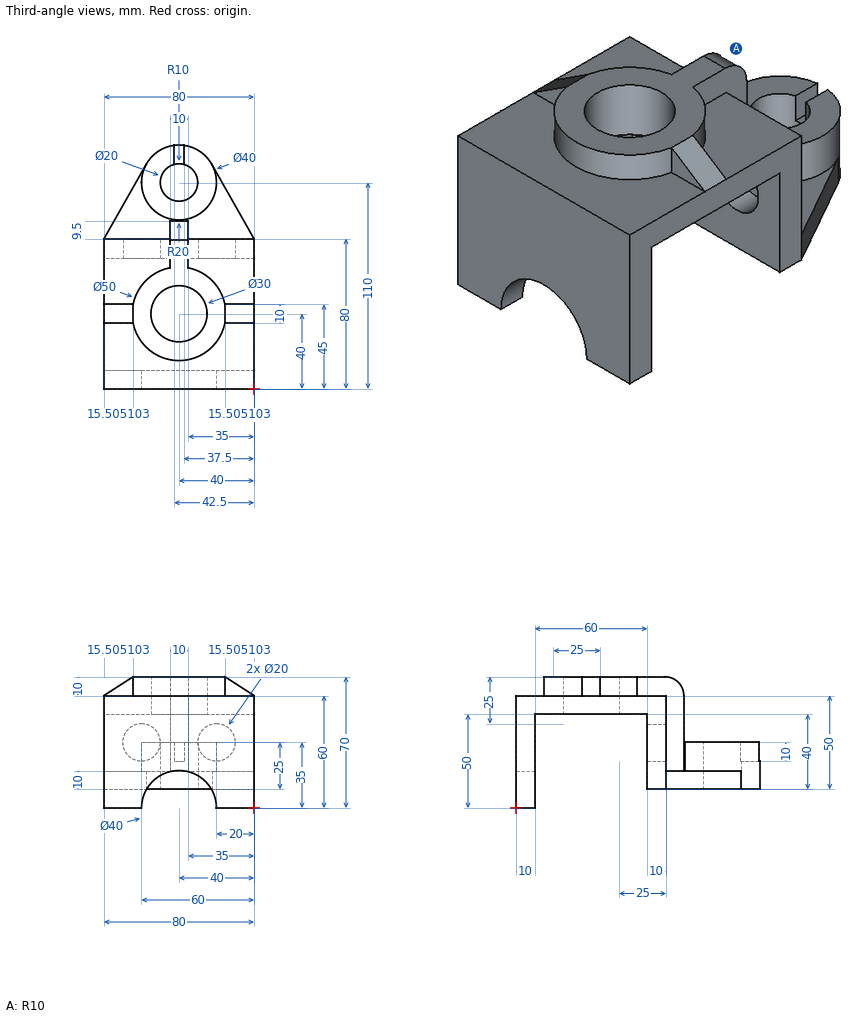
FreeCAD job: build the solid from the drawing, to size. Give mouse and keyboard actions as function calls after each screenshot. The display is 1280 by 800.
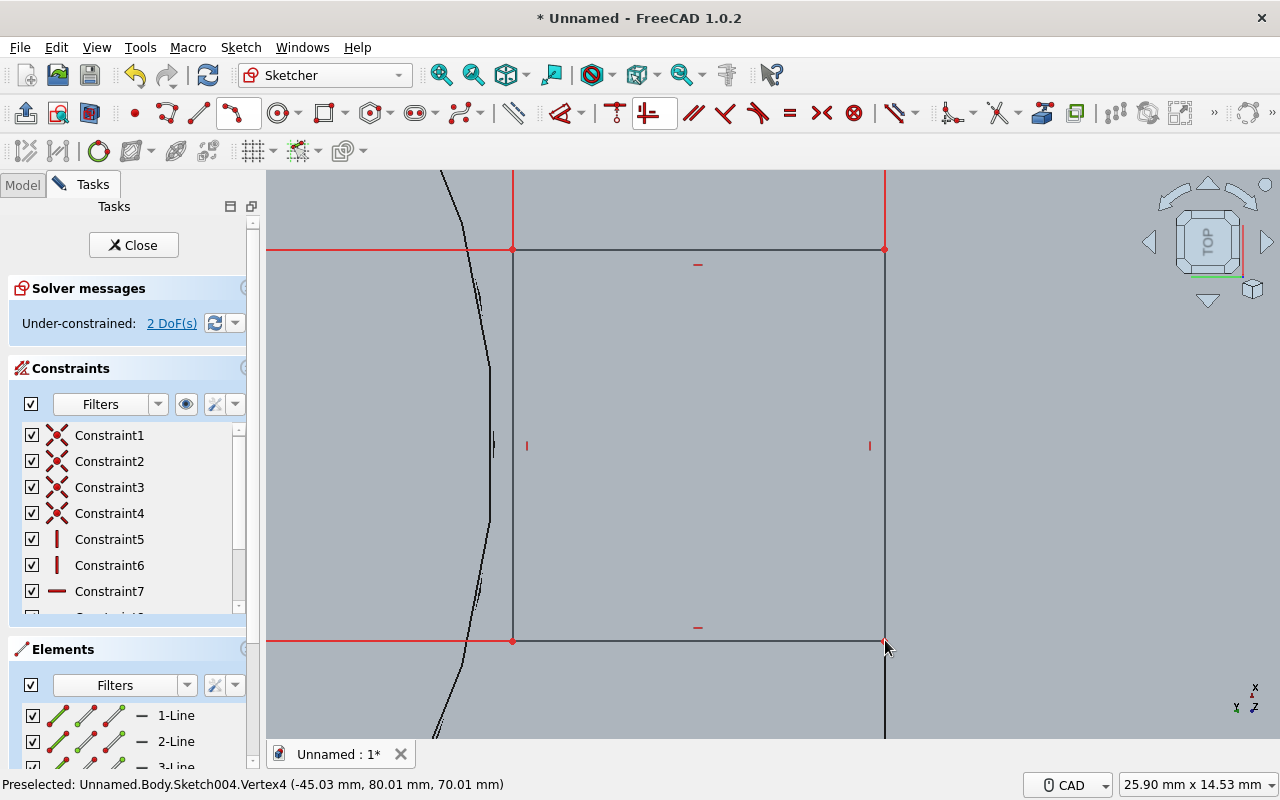
click(560, 114)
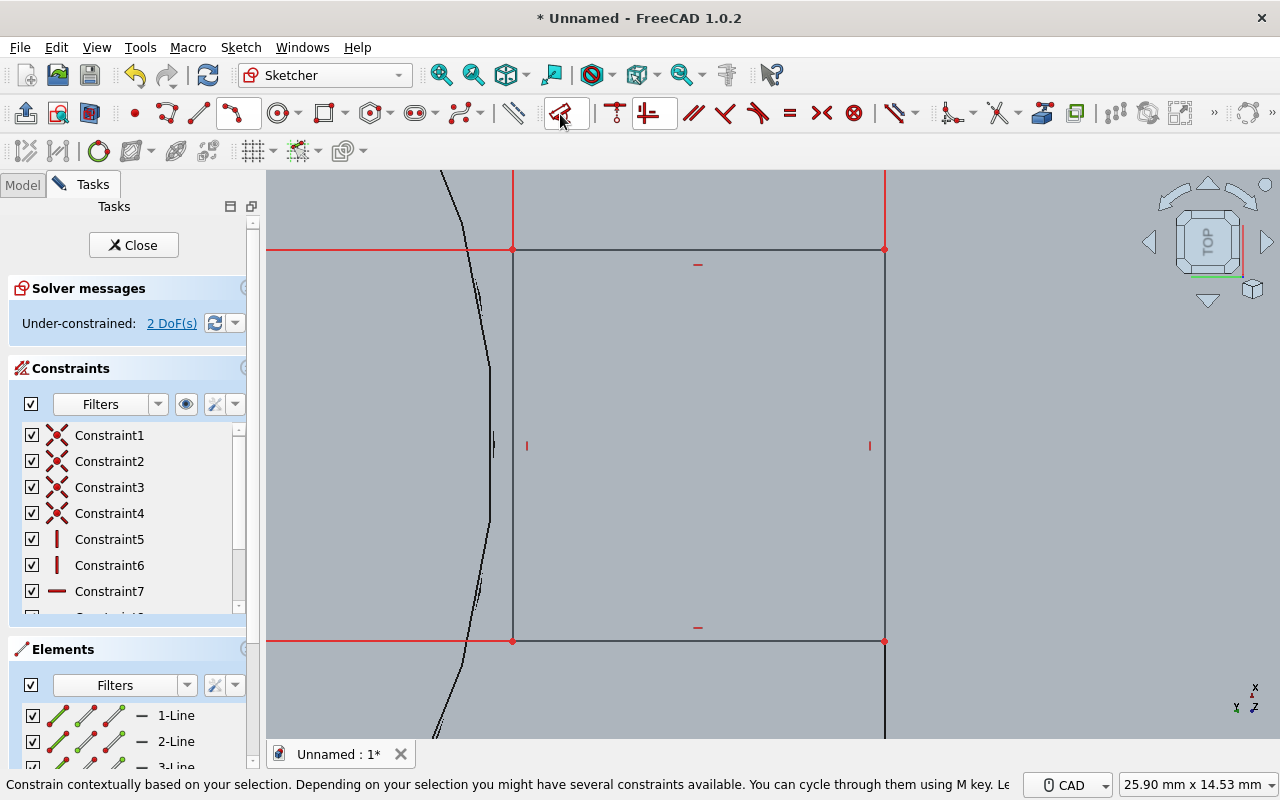
click(513, 250)
click(479, 224)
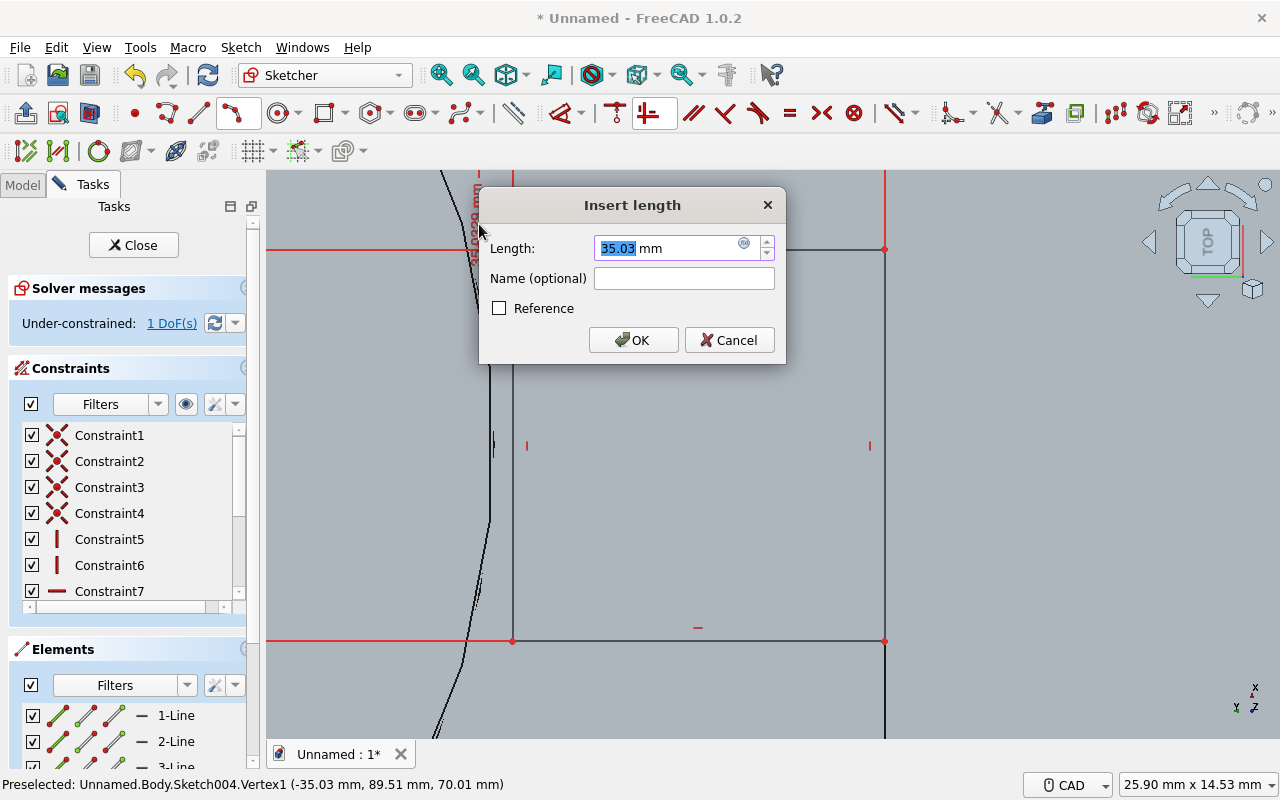
text(35)
key(Return)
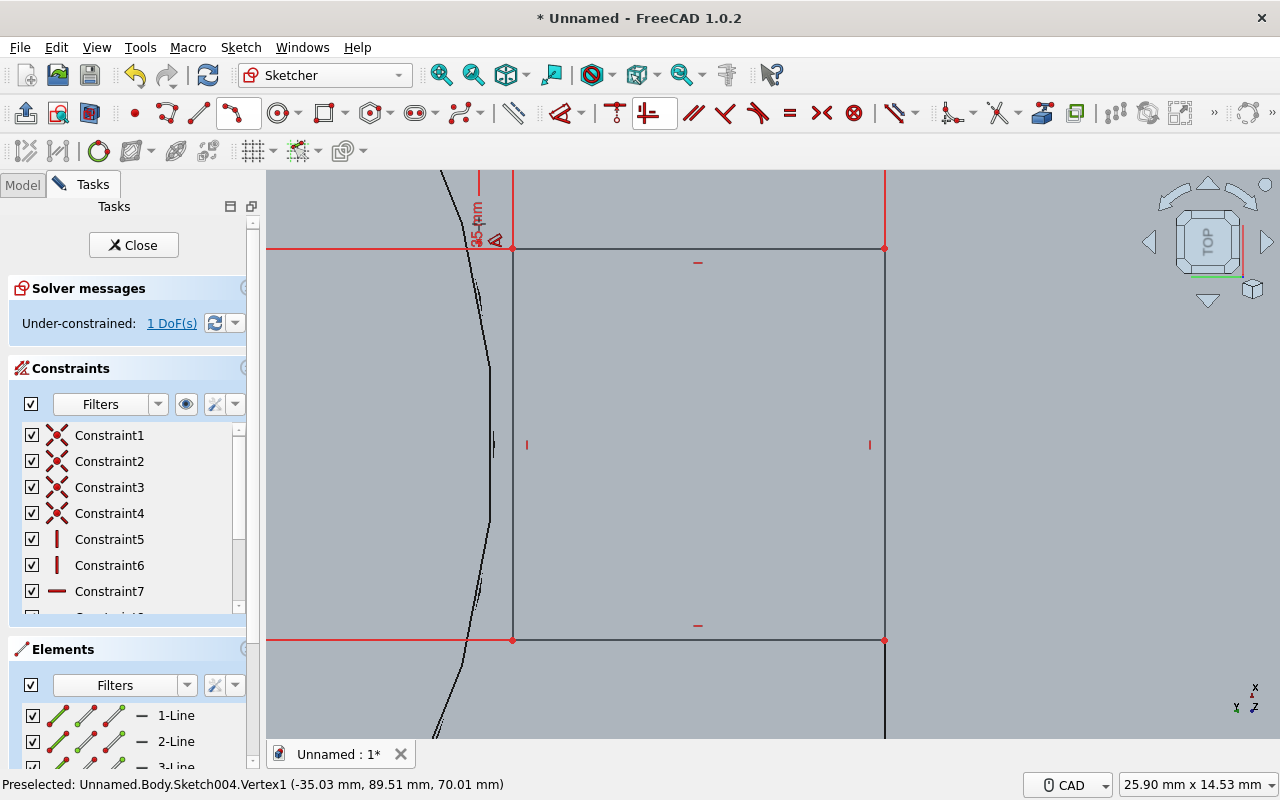
click(885, 640)
click(1000, 674)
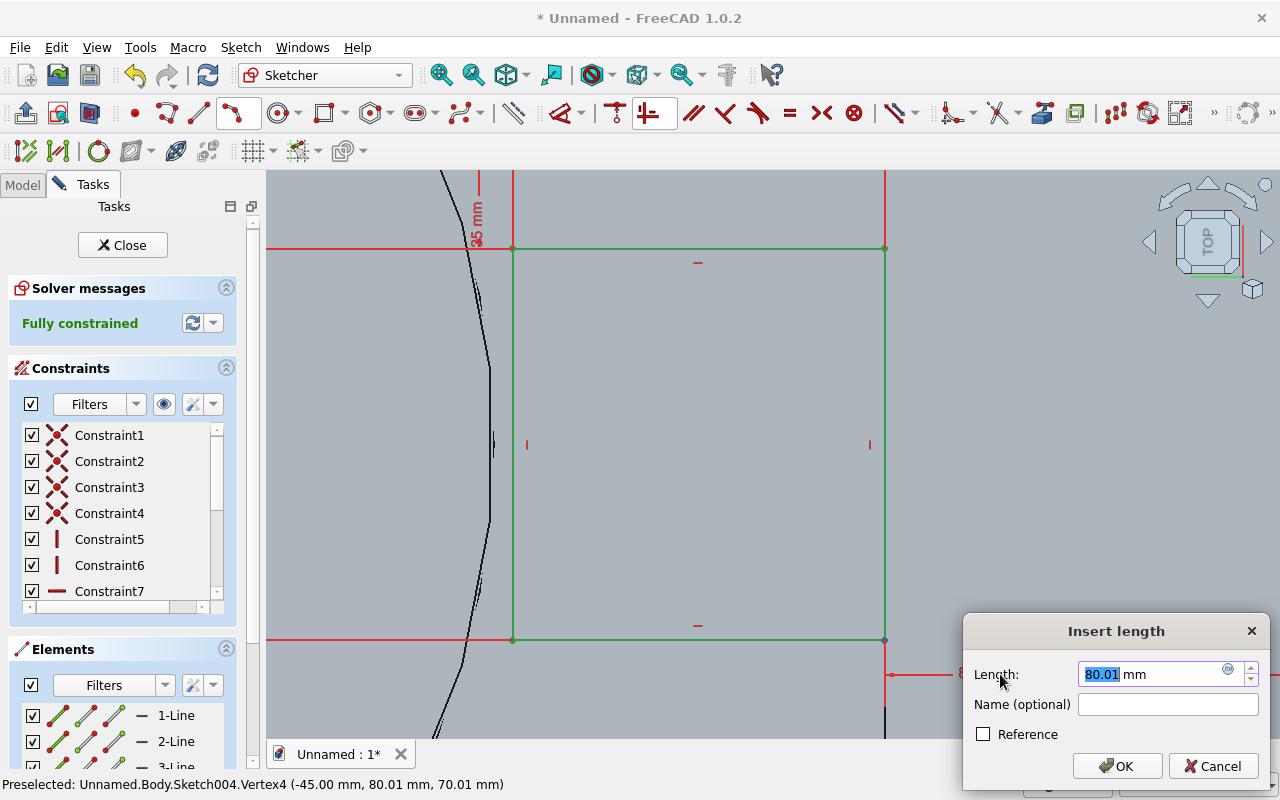
text(80)
key(Return)
key(Escape)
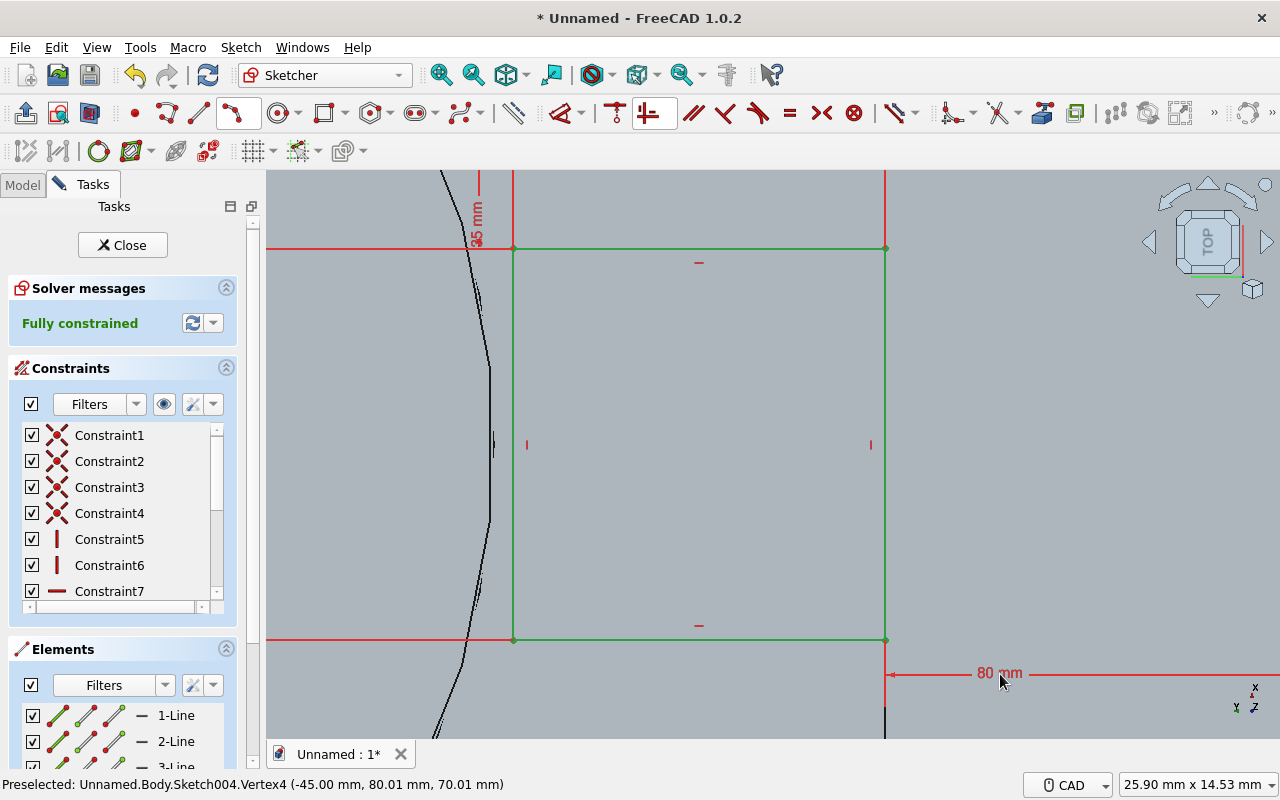
click(123, 245)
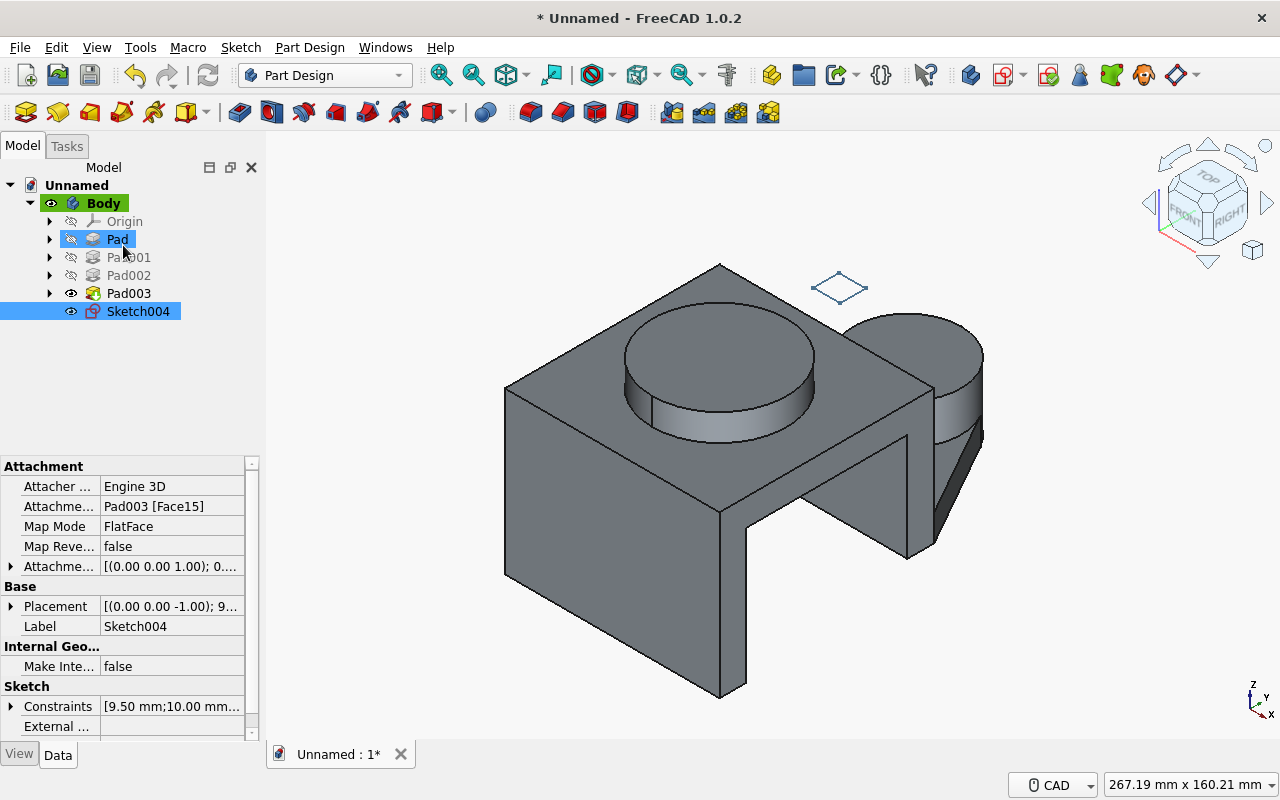
click(26, 112)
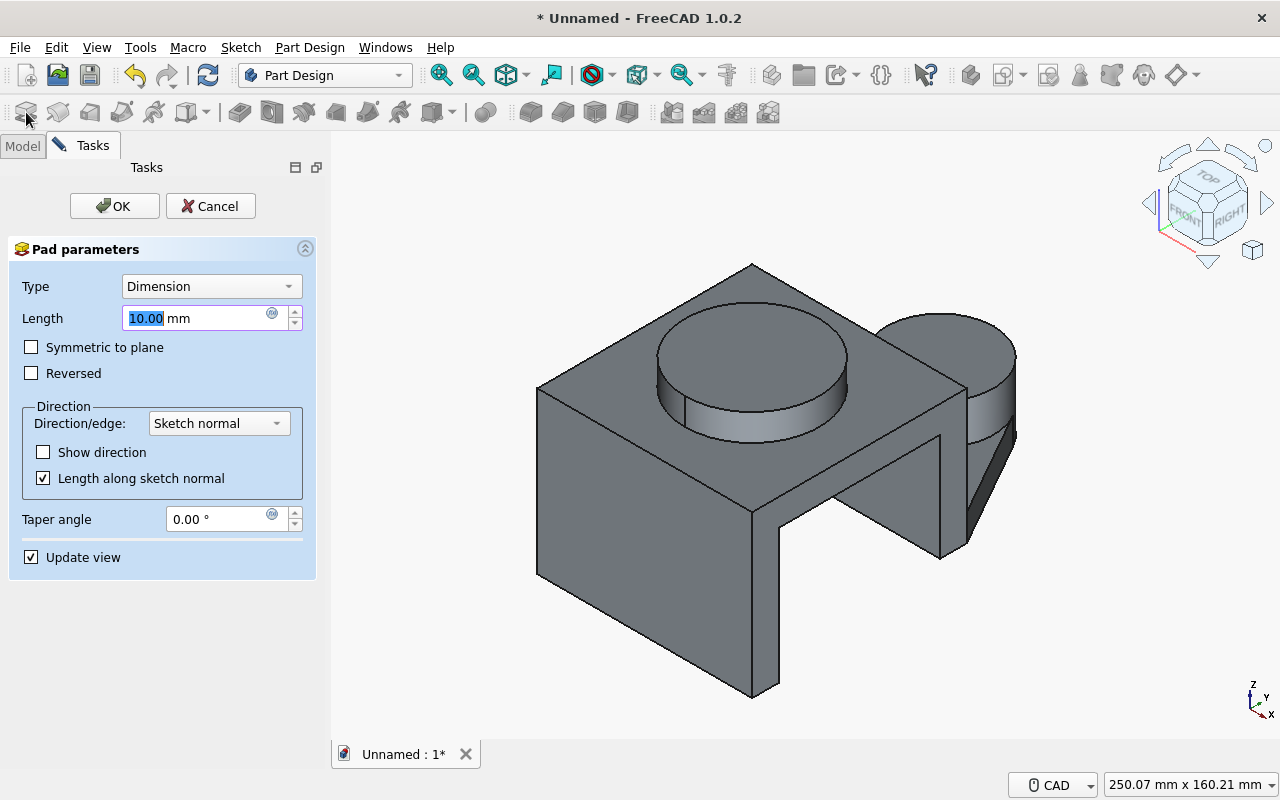
click(212, 286)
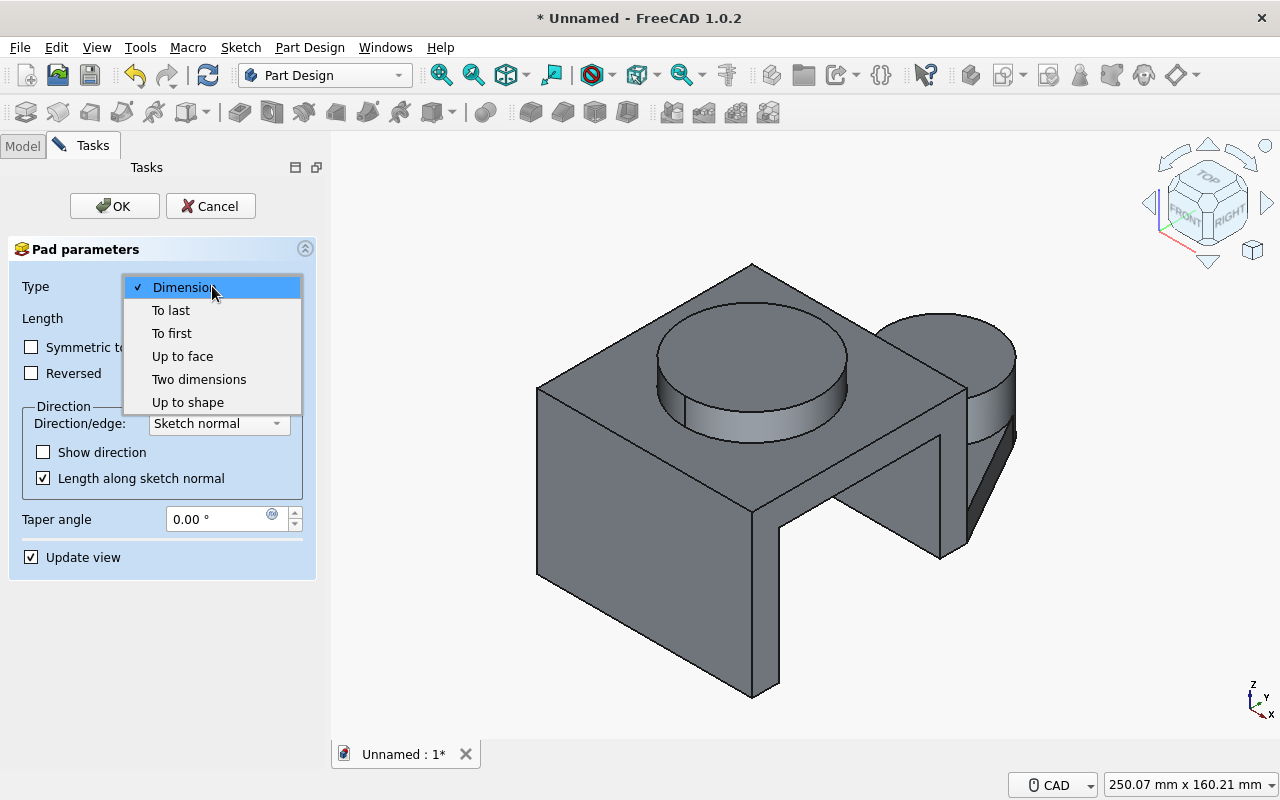
click(212, 334)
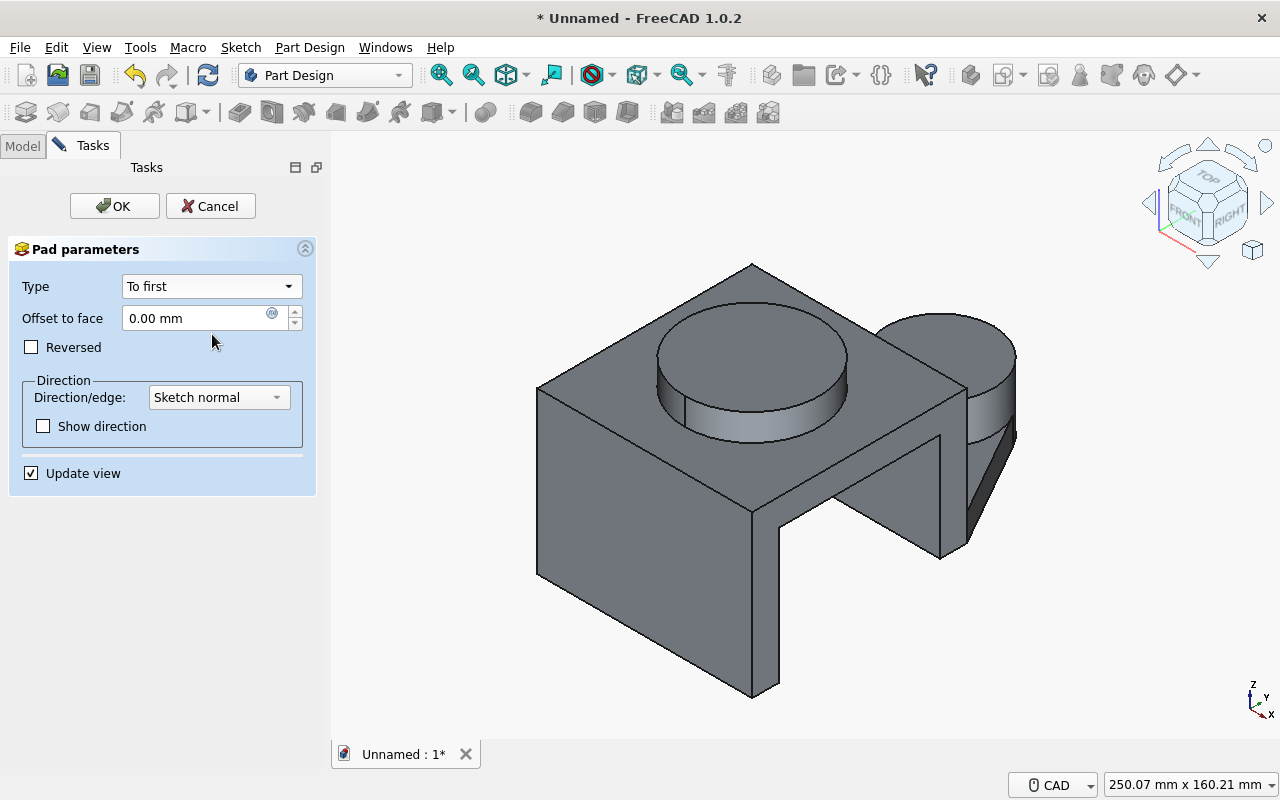
click(30, 347)